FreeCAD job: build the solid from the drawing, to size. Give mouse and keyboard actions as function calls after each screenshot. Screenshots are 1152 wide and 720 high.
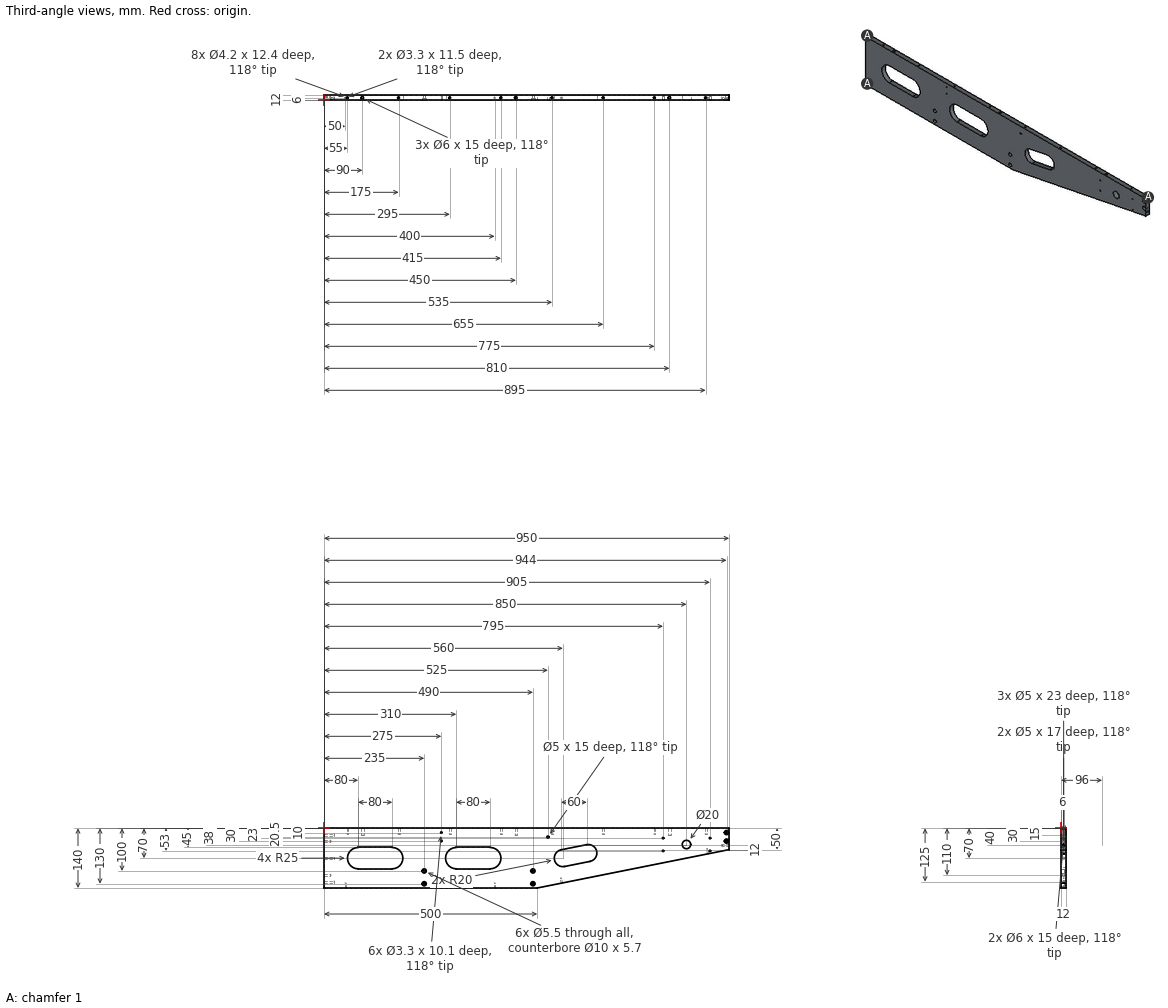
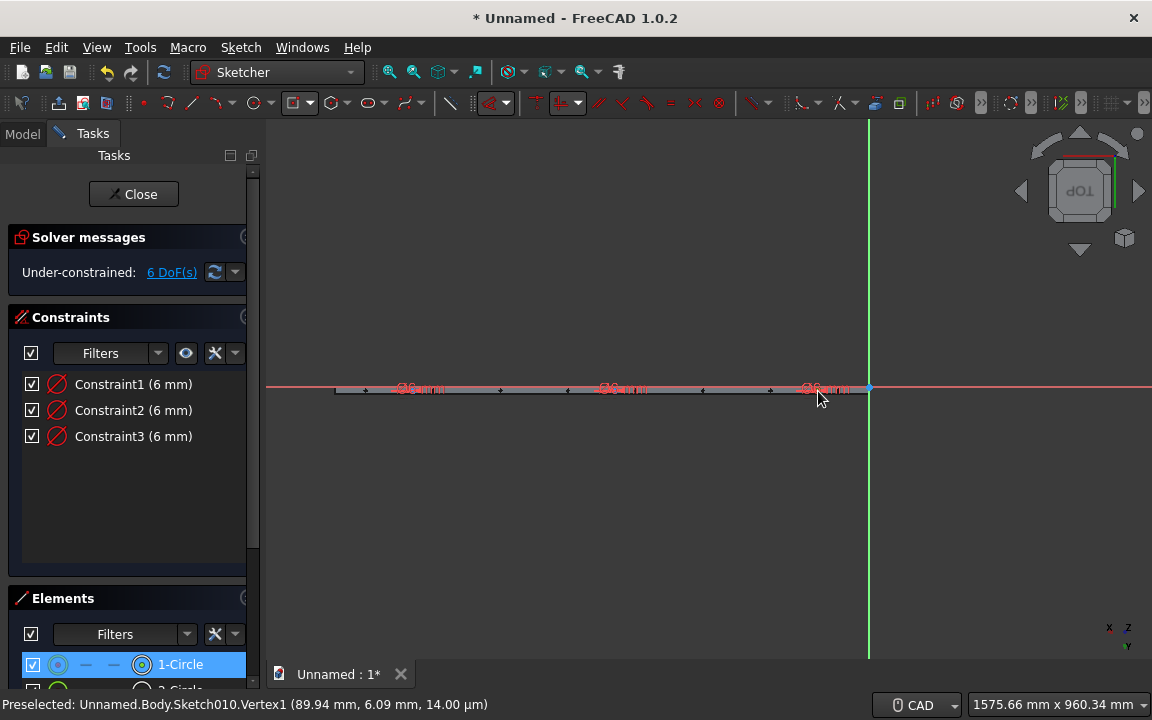
click(616, 391)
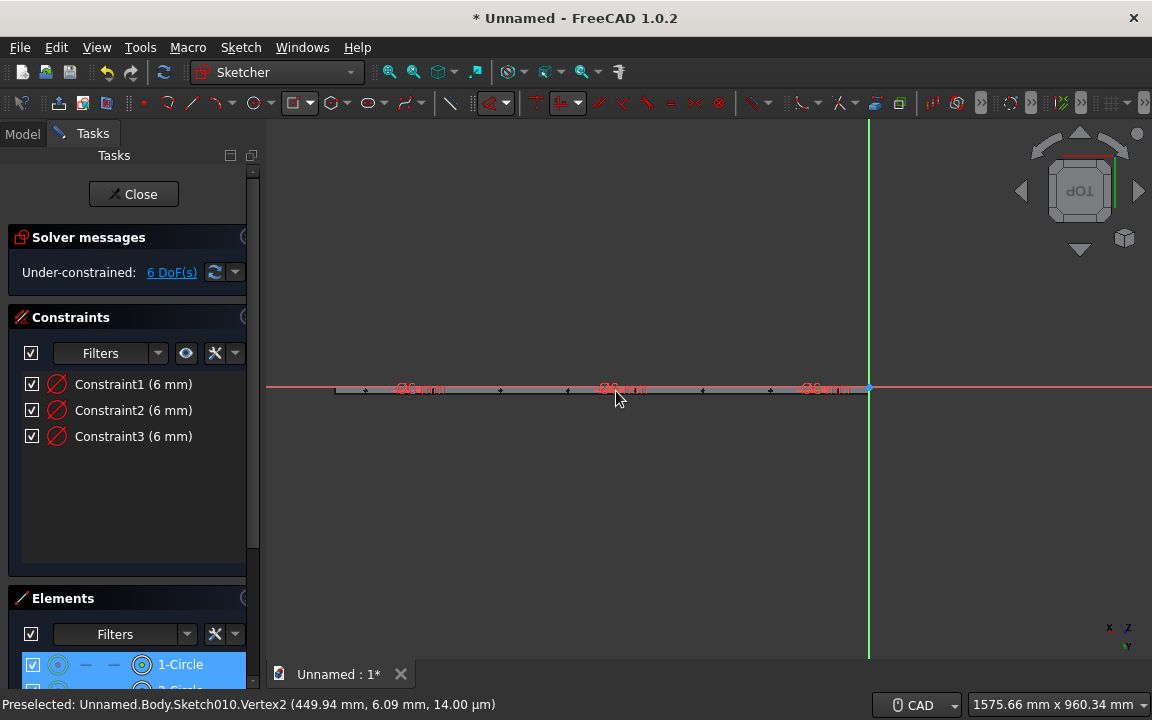
key(h)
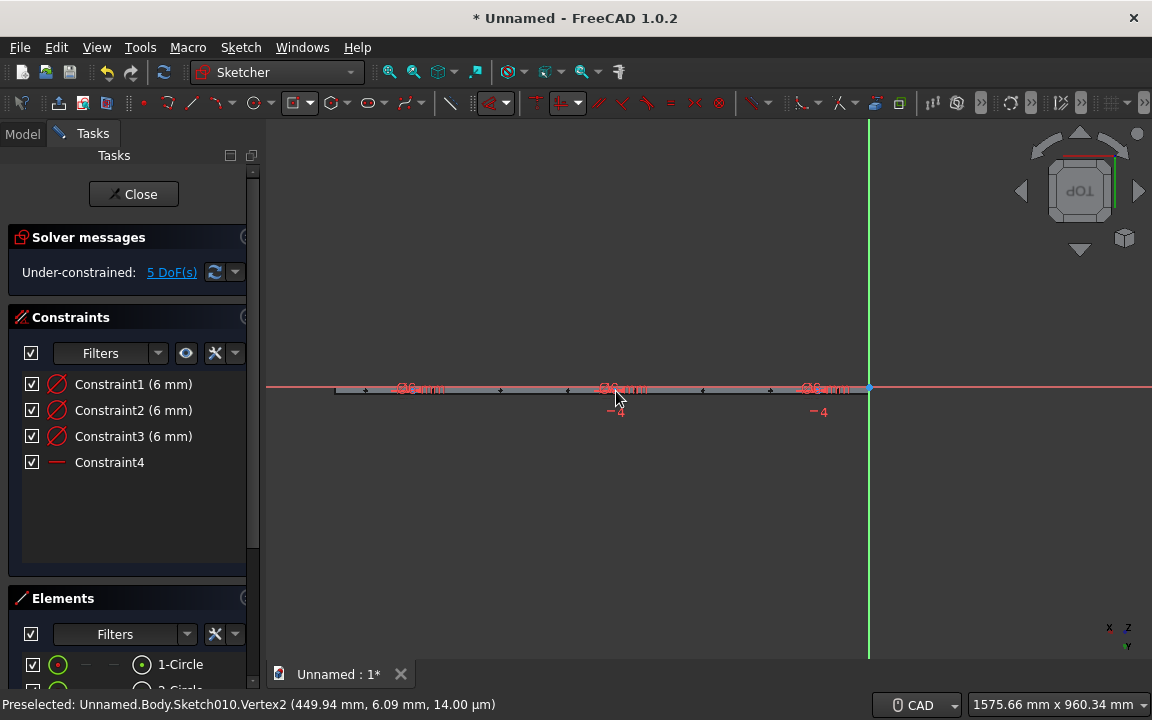
click(616, 391)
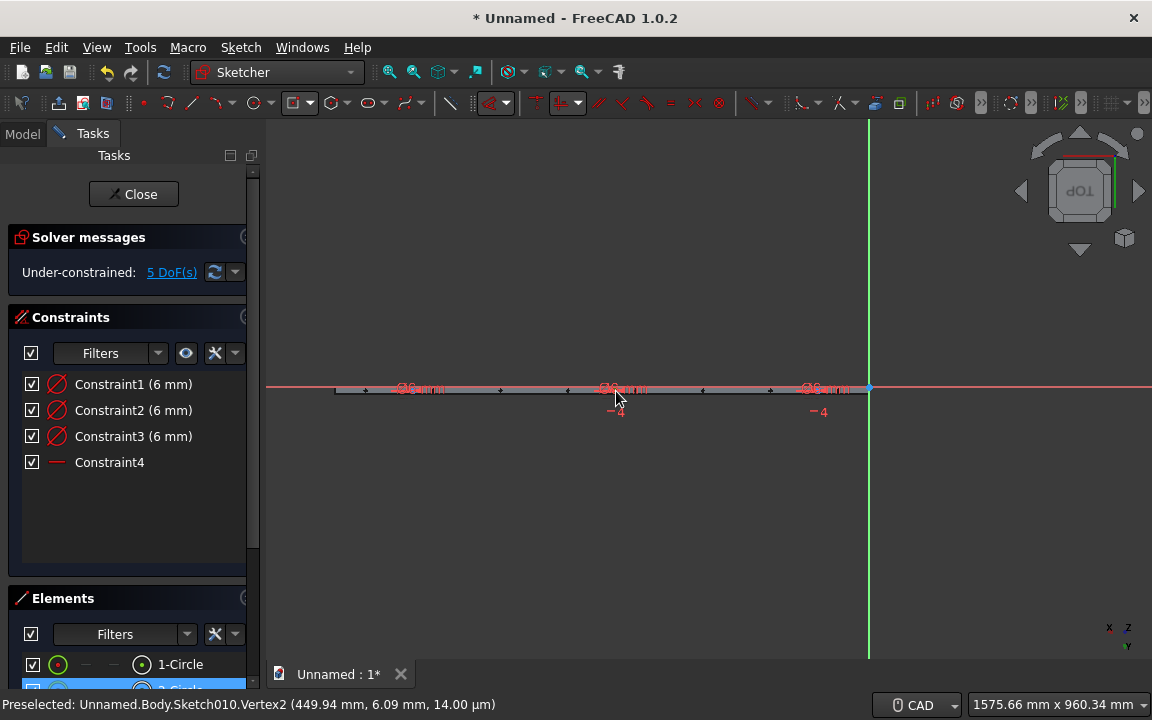
click(414, 391)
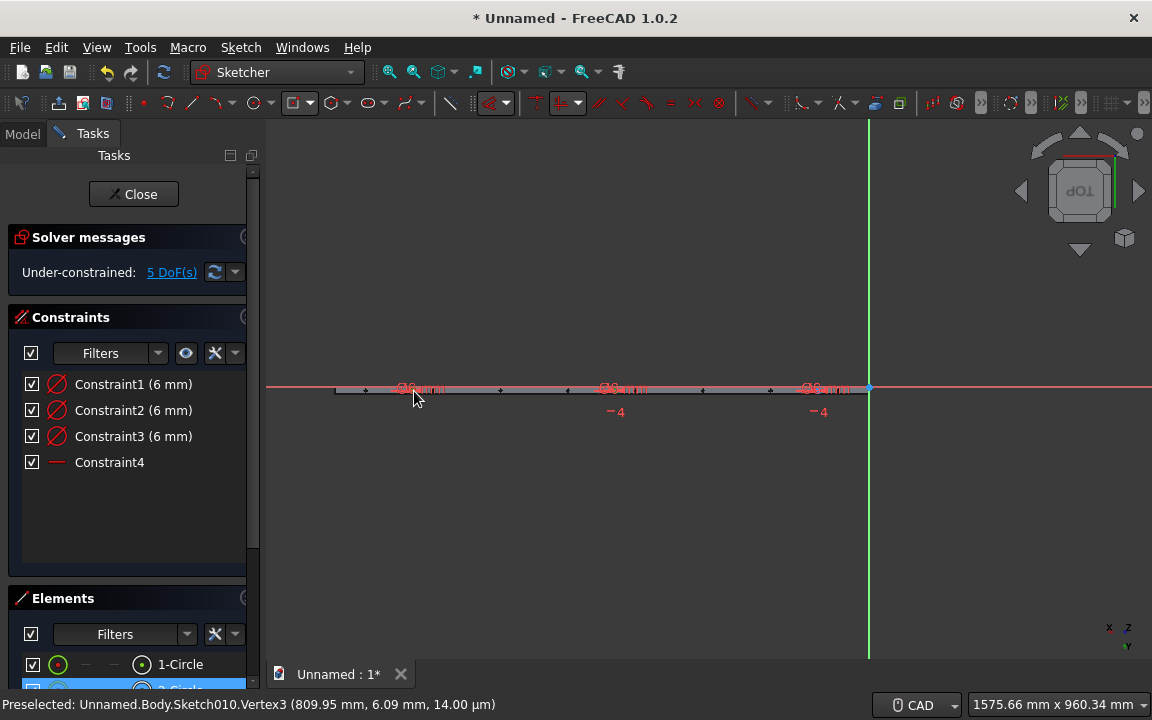
key(h)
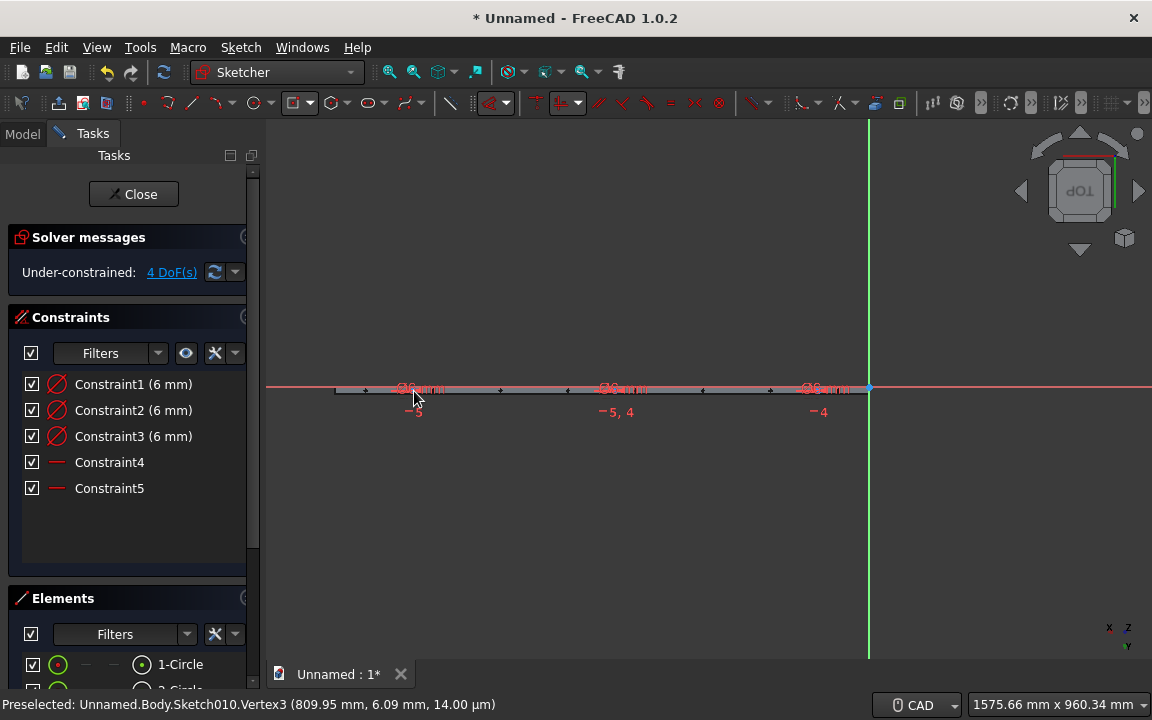
scroll(818, 391, up, 13)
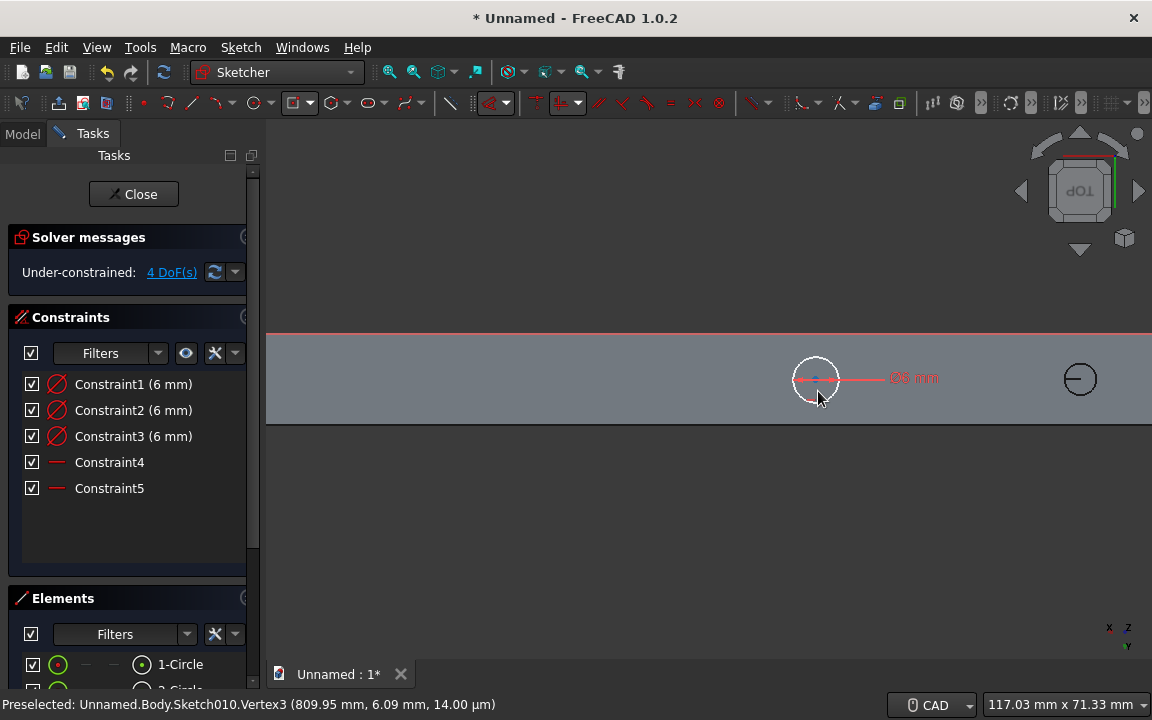
click(816, 380)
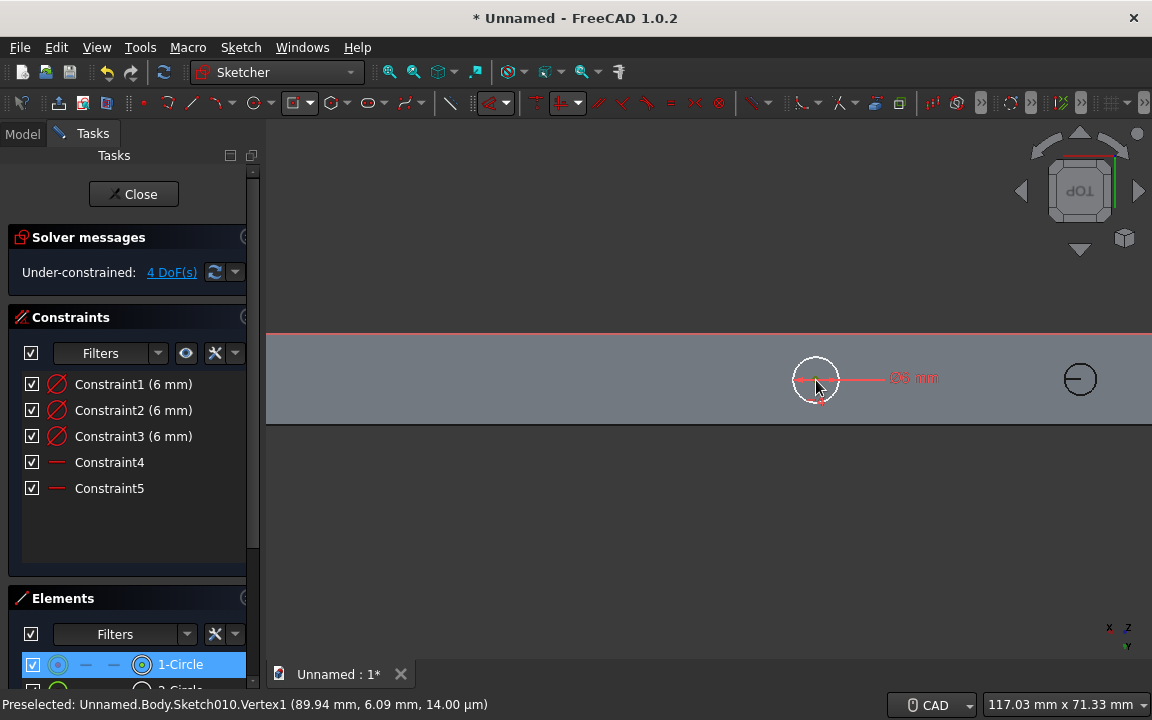
key(i)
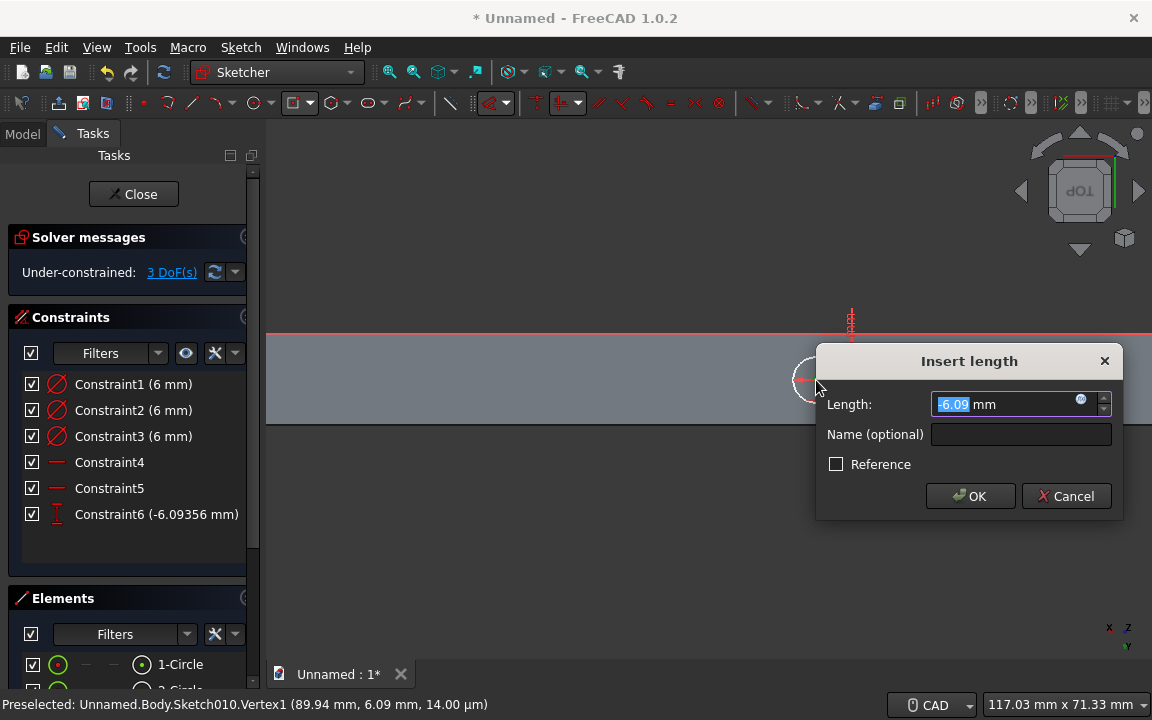
text(-6)
key(Return)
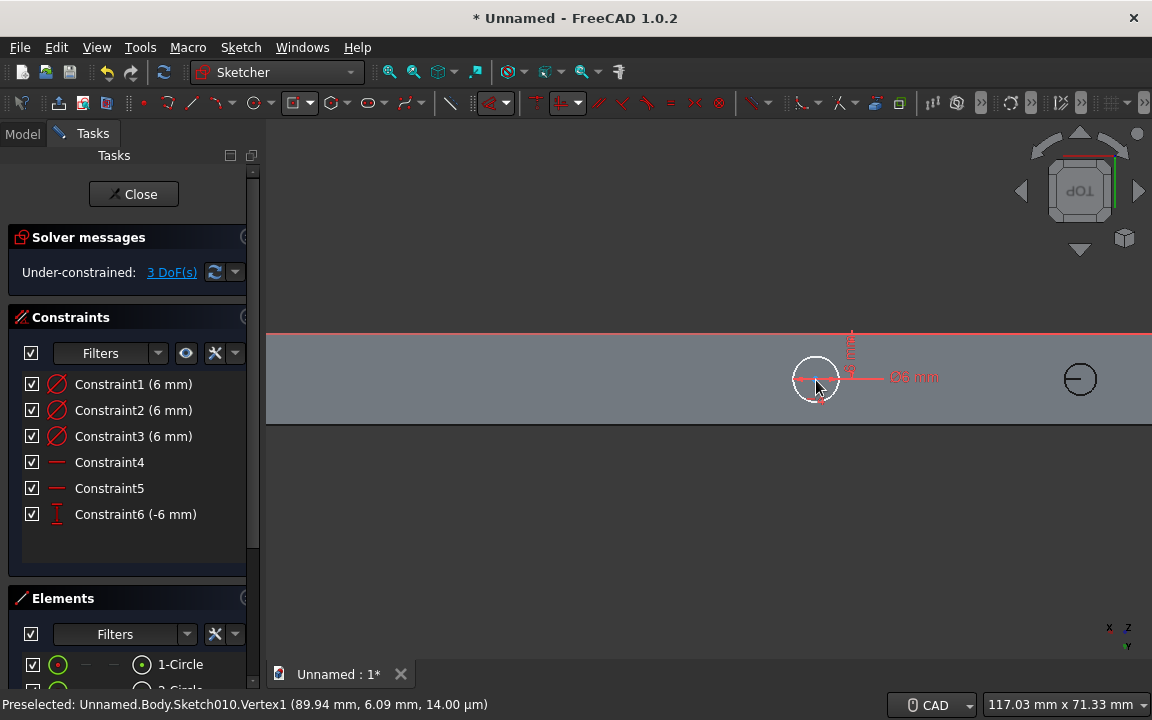
scroll(819, 391, down, 13)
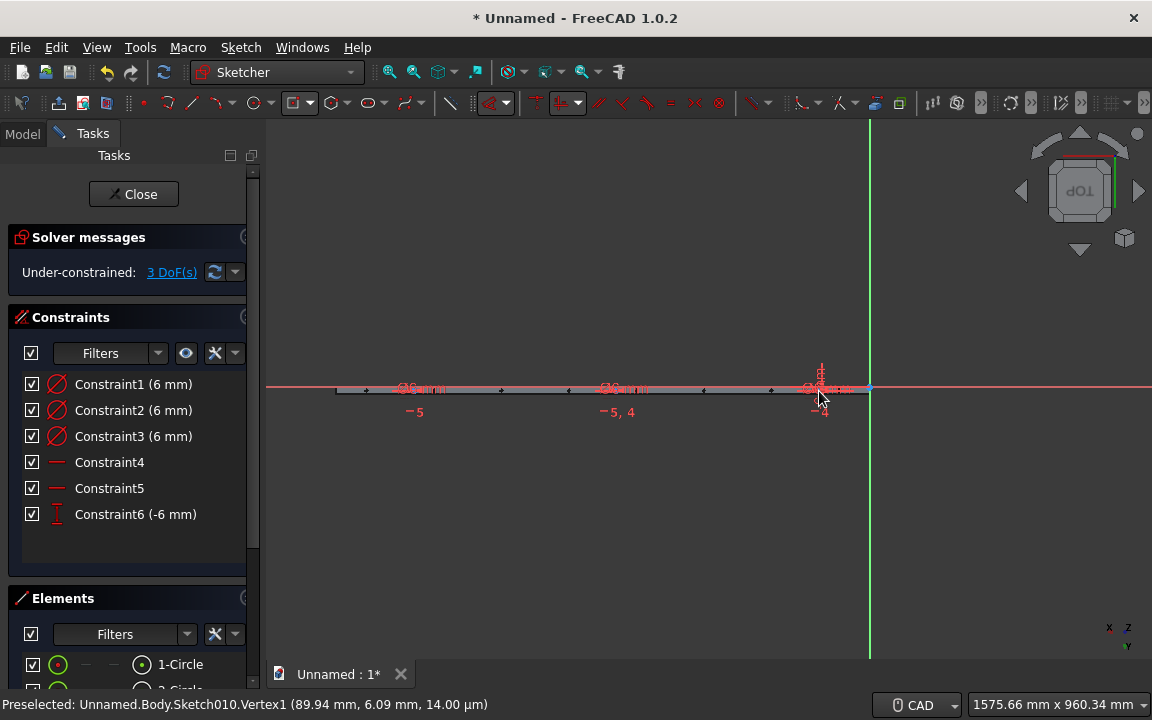
click(819, 391)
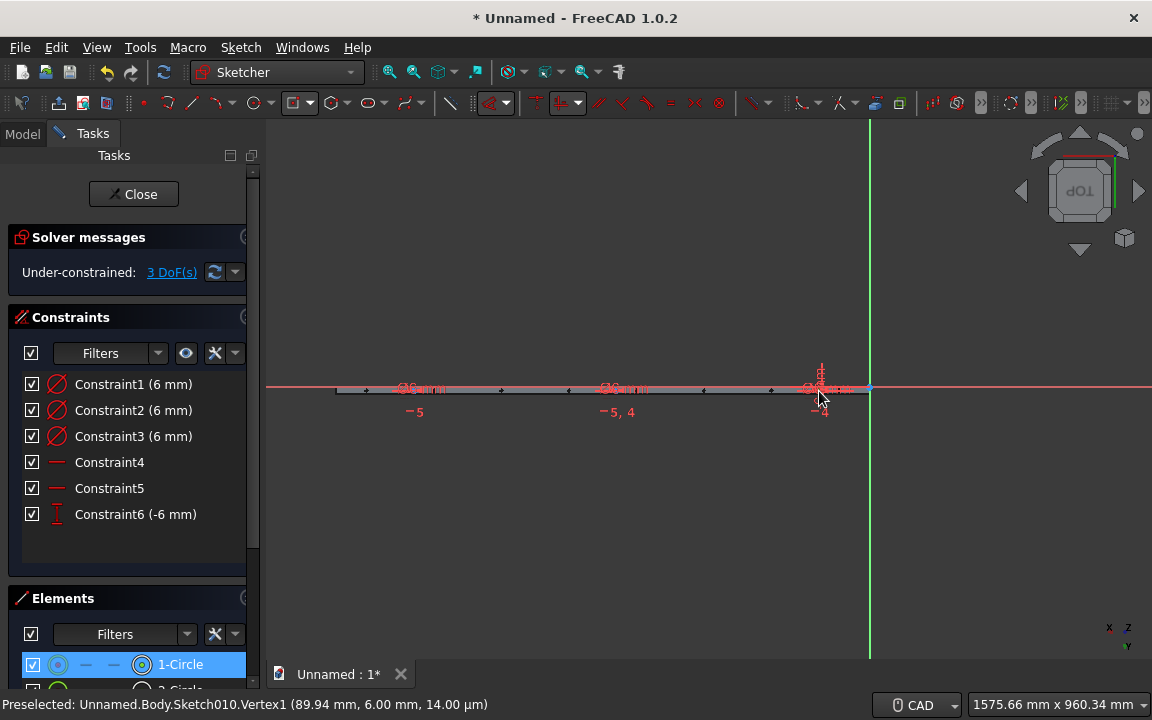
key(l)